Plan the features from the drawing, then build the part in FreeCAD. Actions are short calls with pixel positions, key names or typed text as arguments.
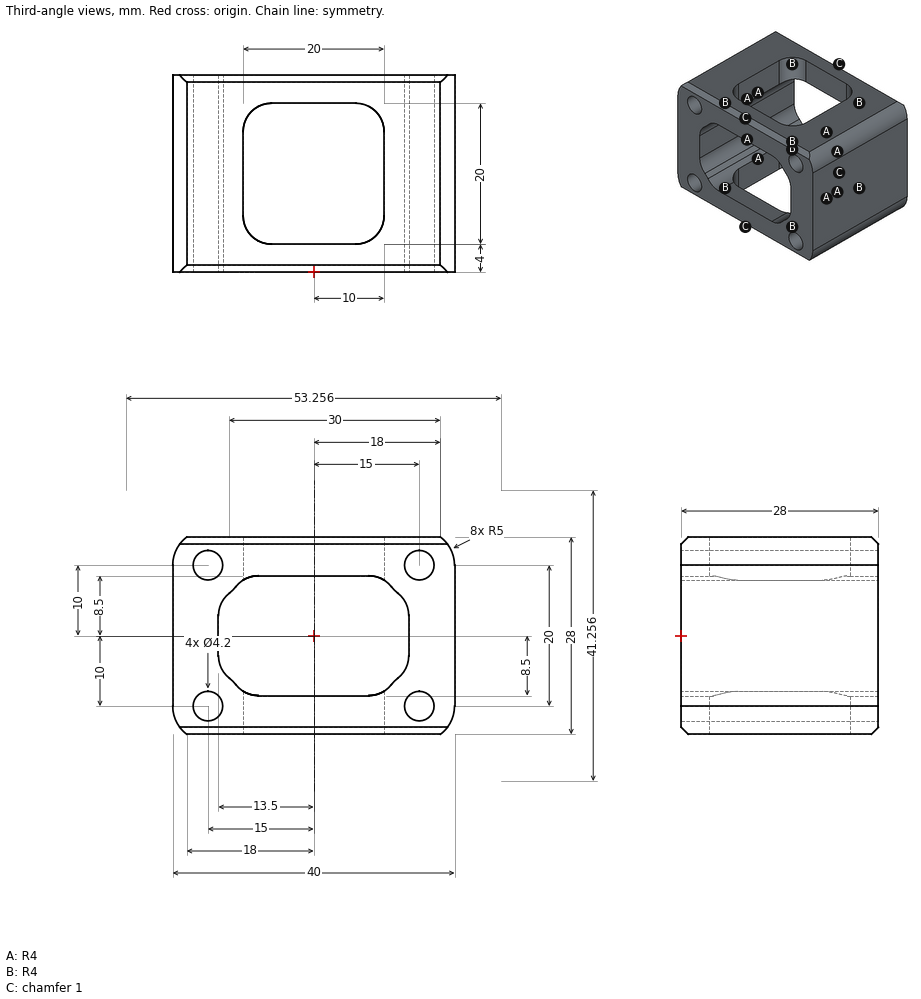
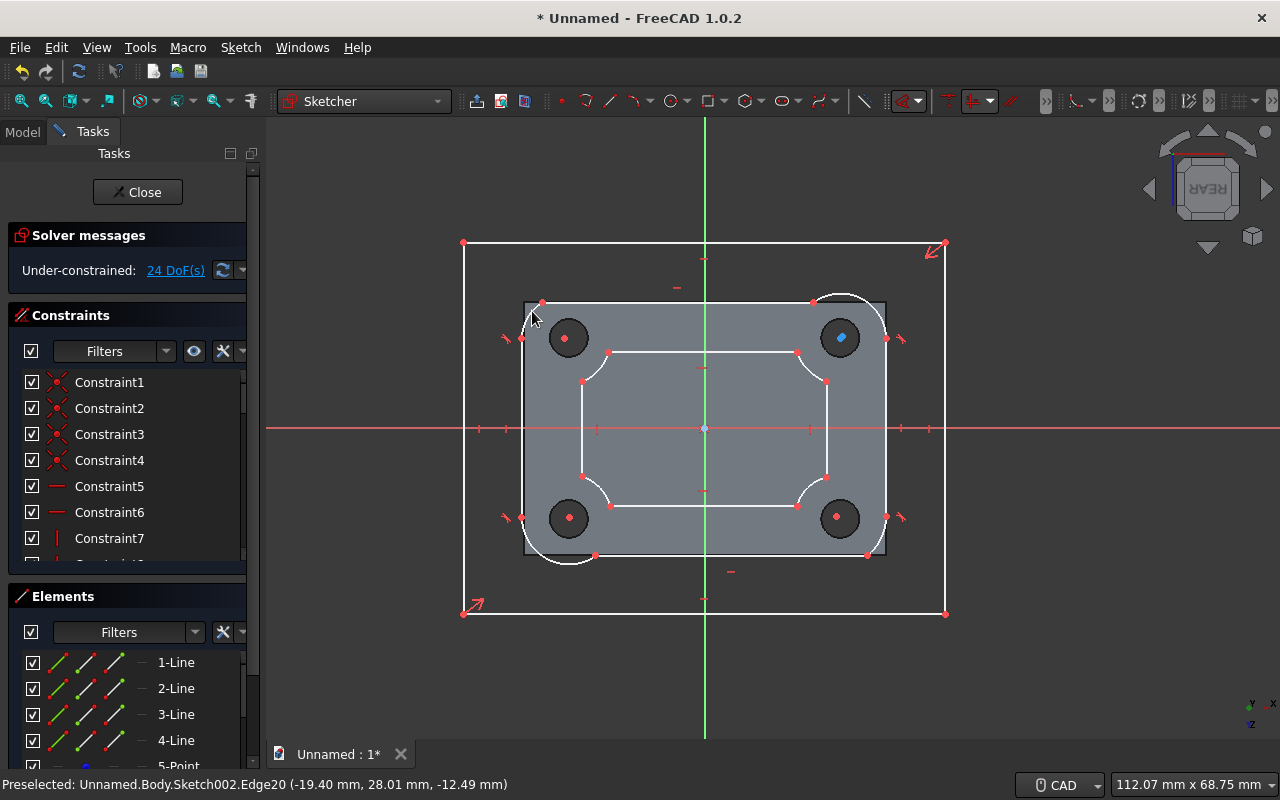
click(803, 364)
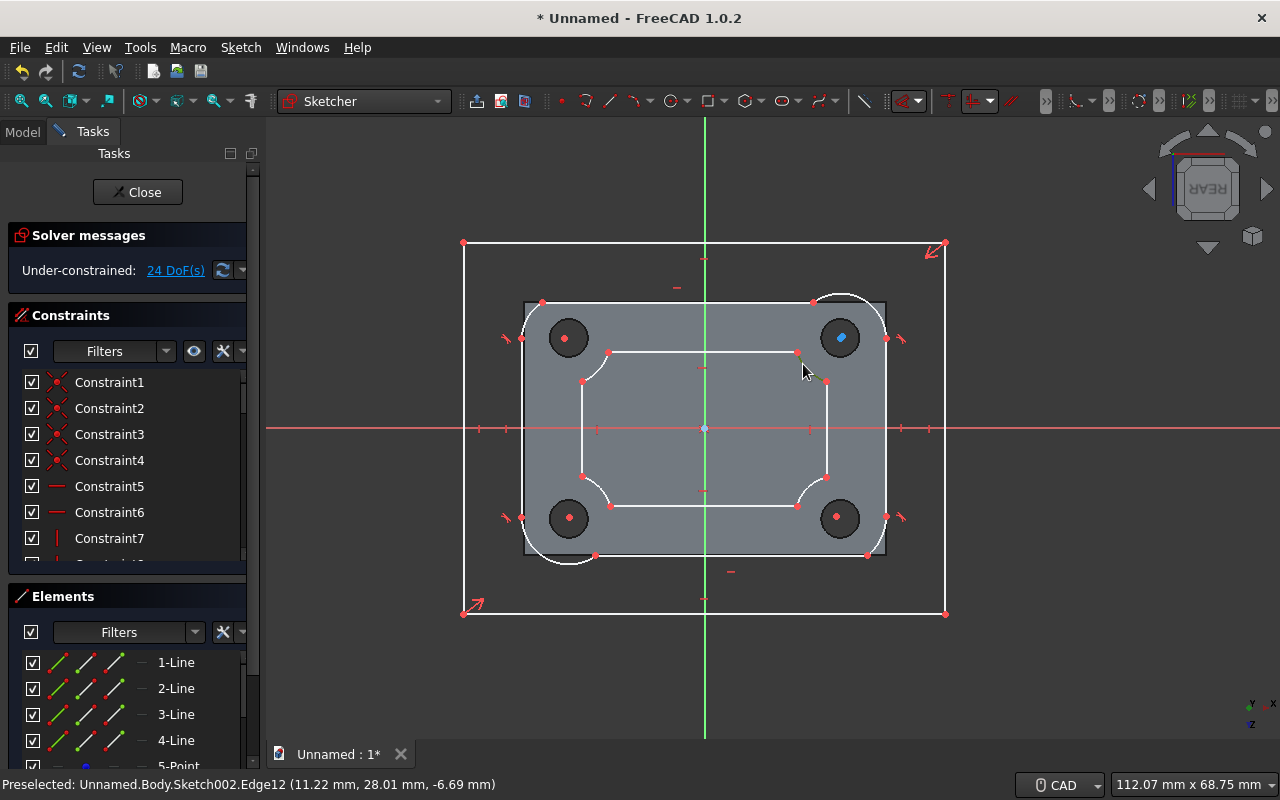
click(876, 311)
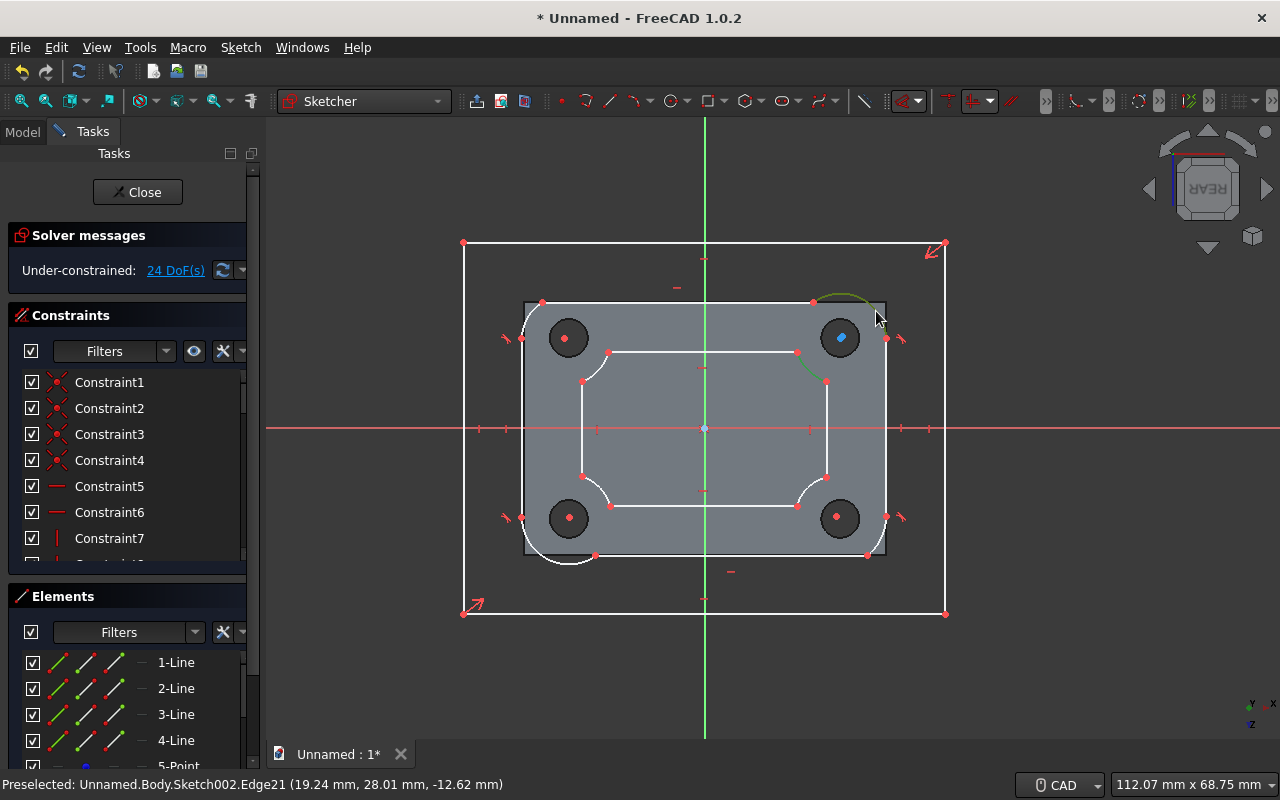
click(948, 102)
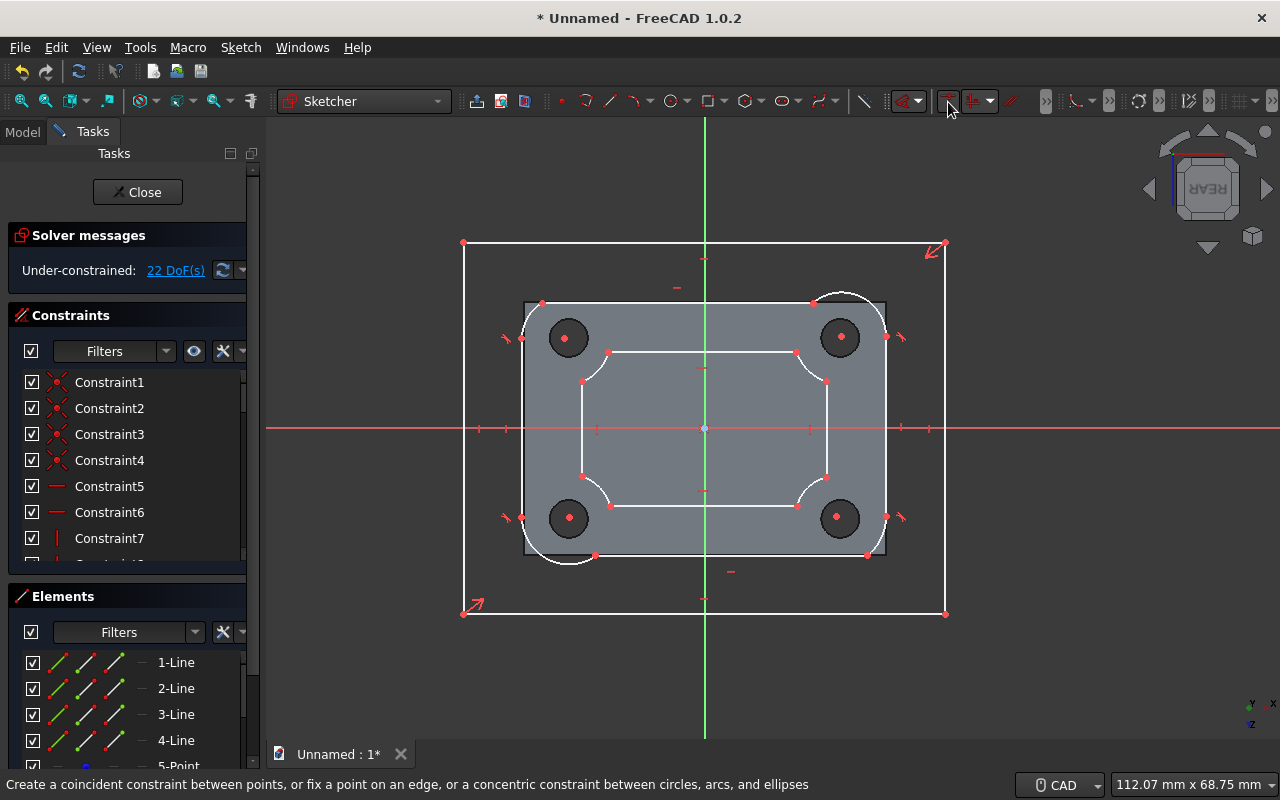
click(605, 495)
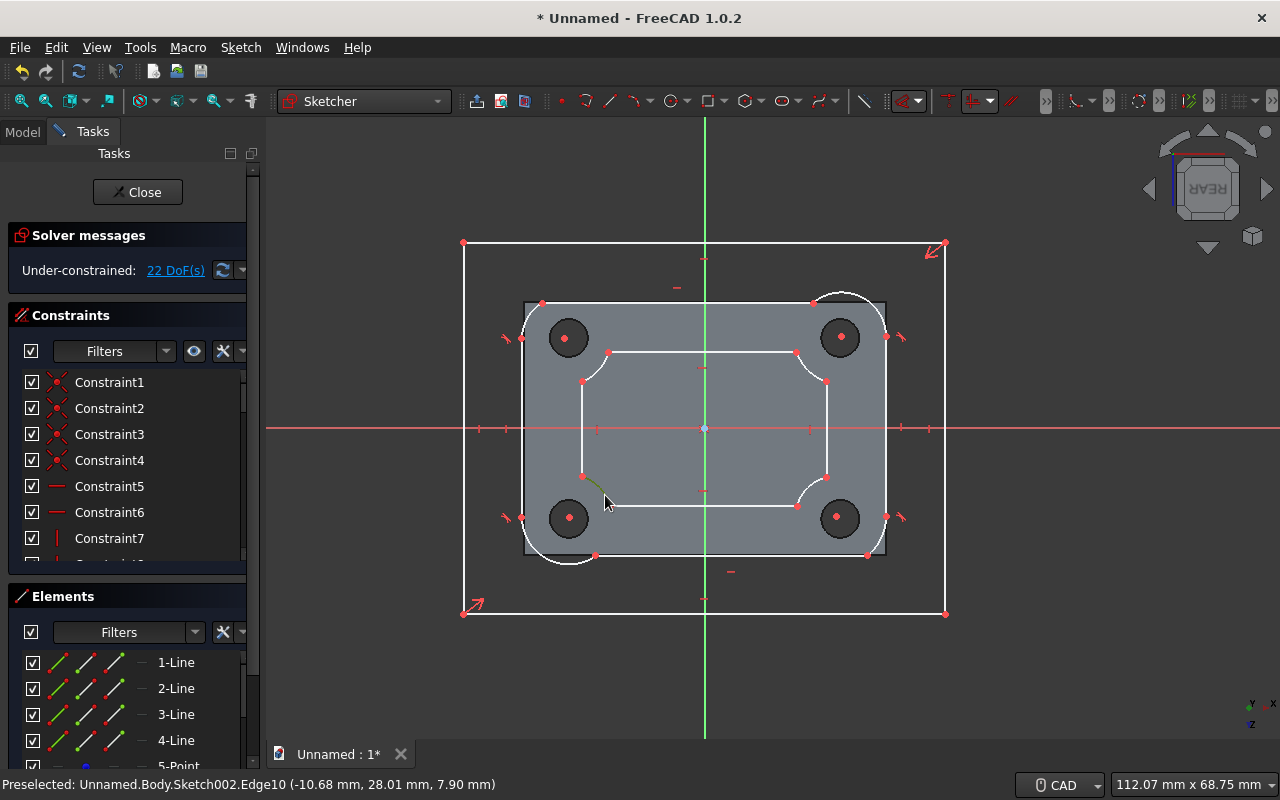
click(815, 482)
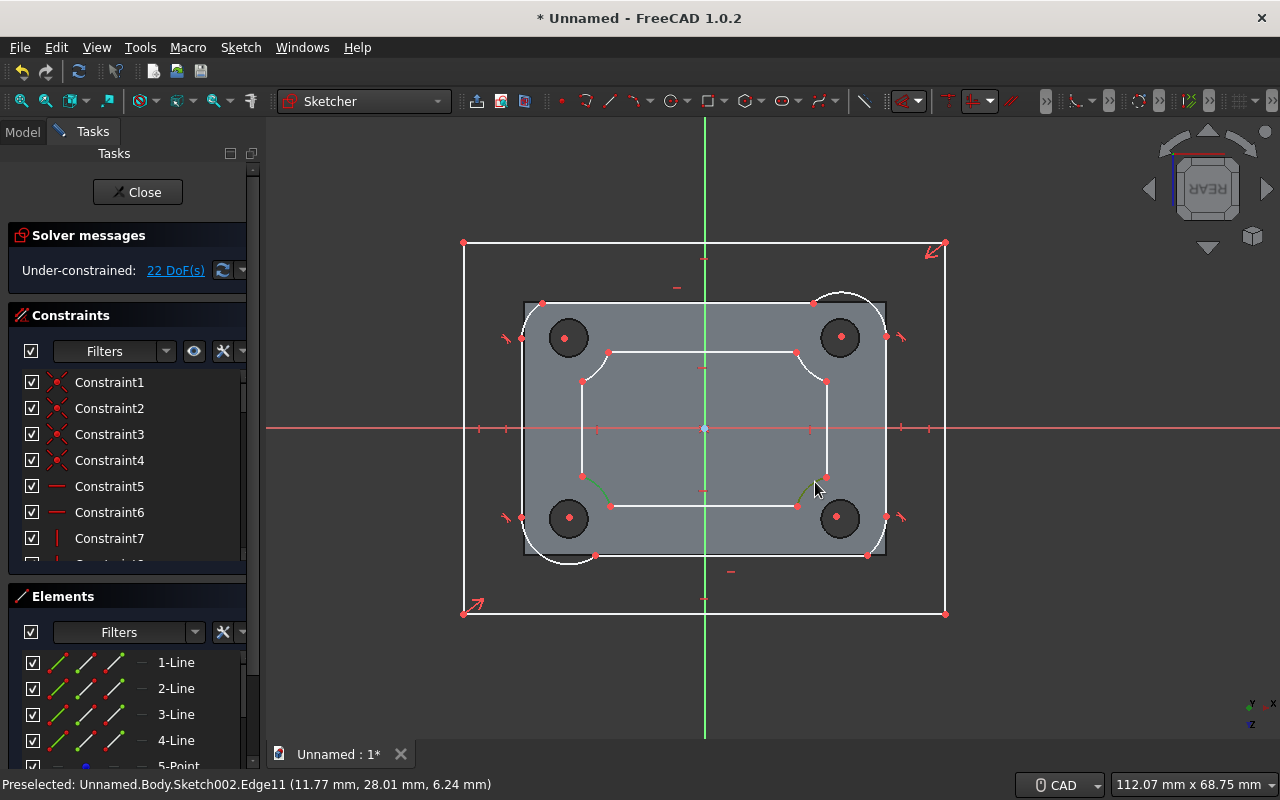
click(803, 364)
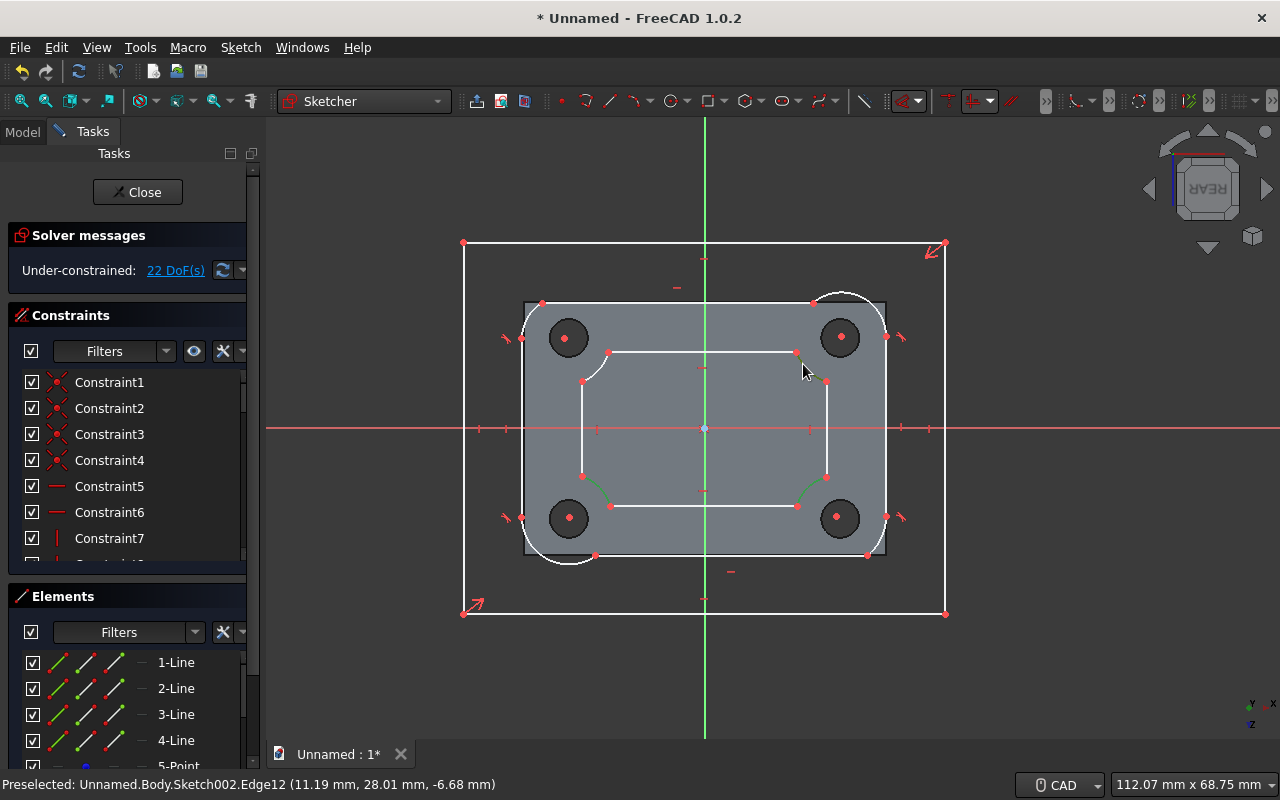
click(593, 376)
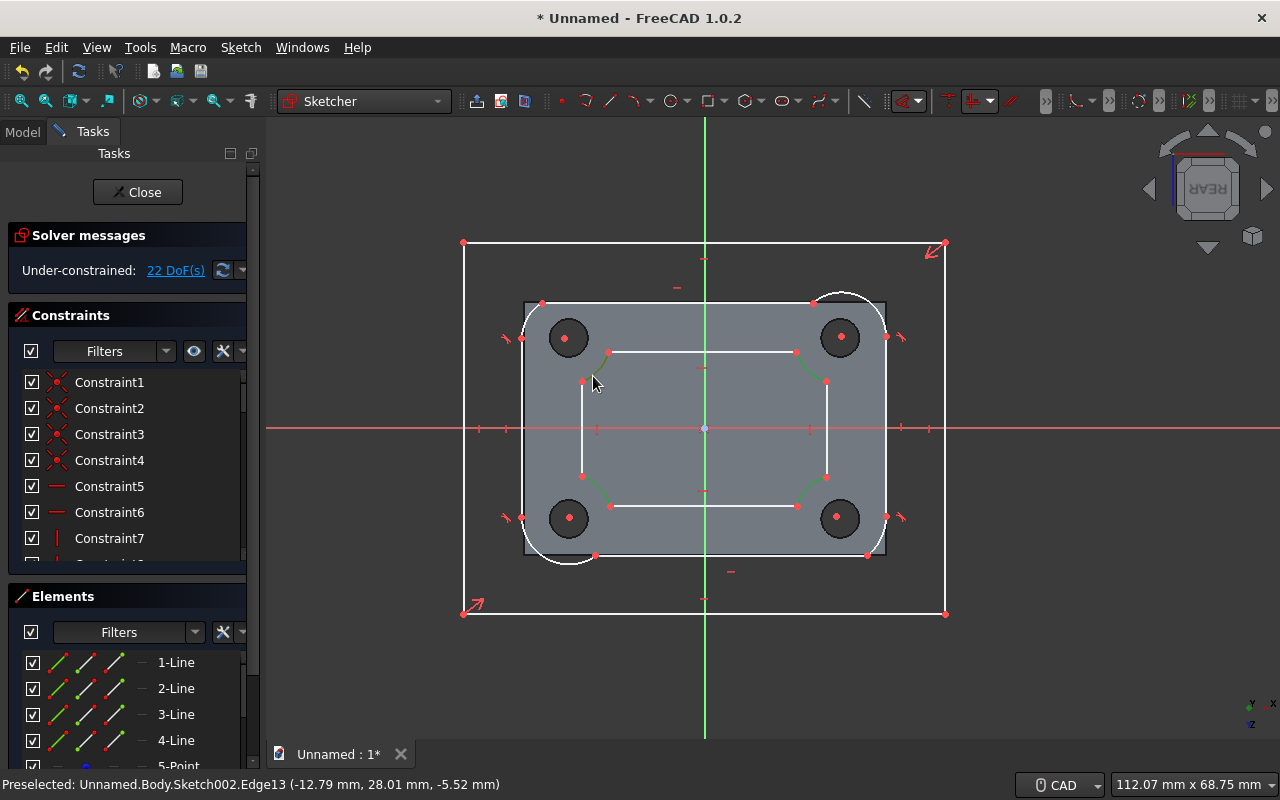
click(876, 546)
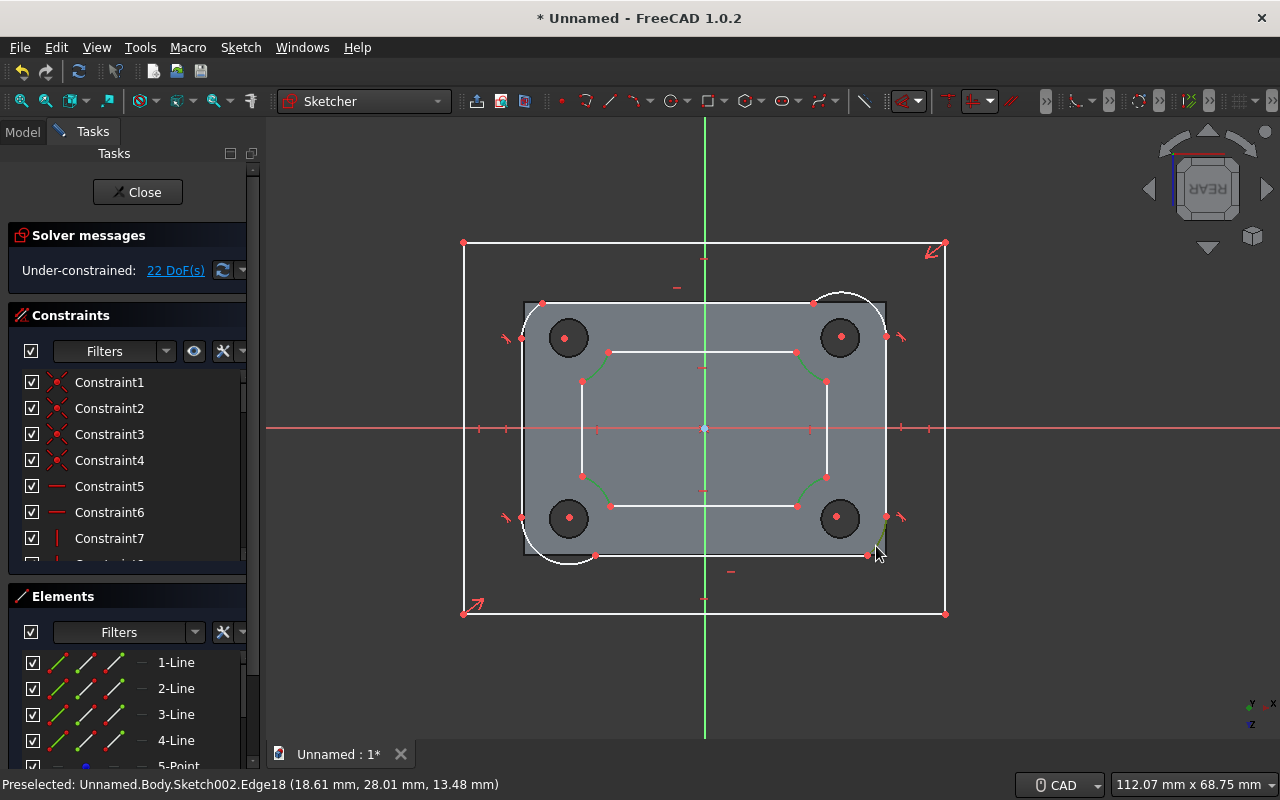
click(532, 546)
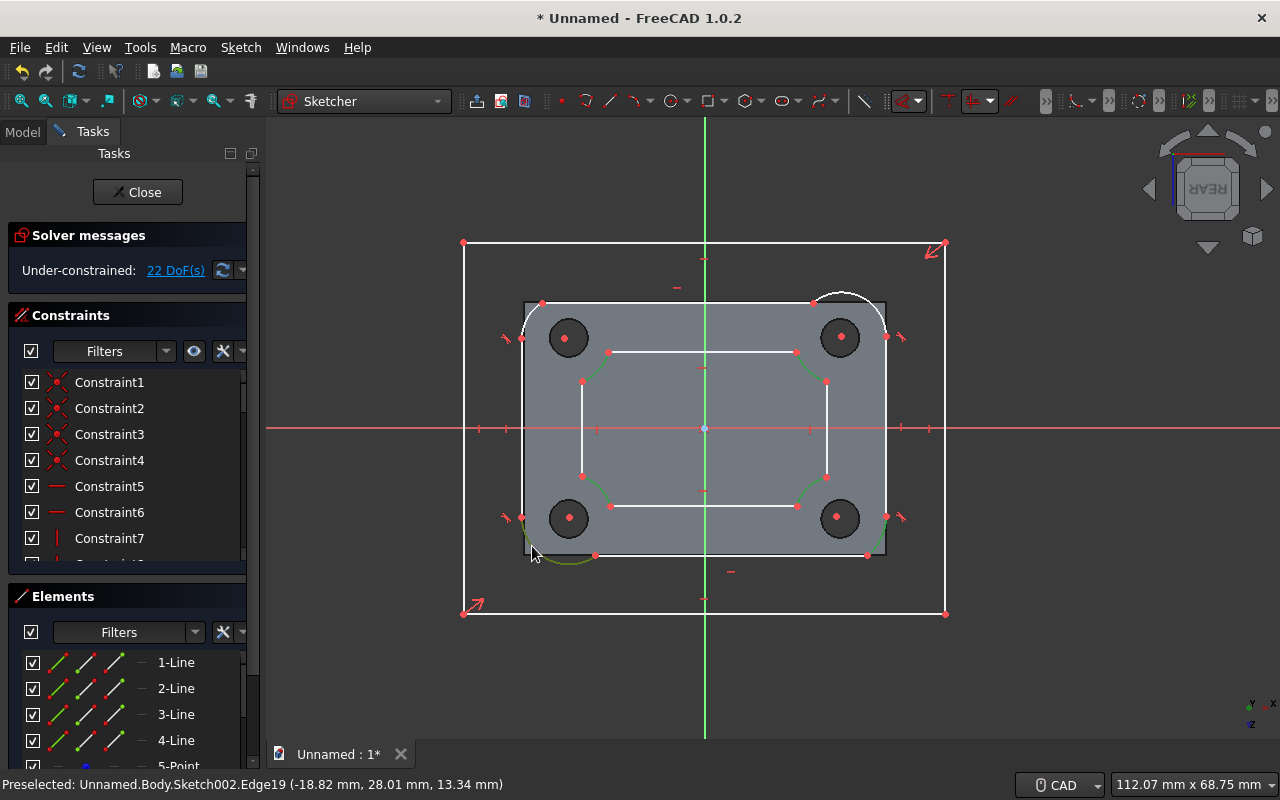
click(532, 311)